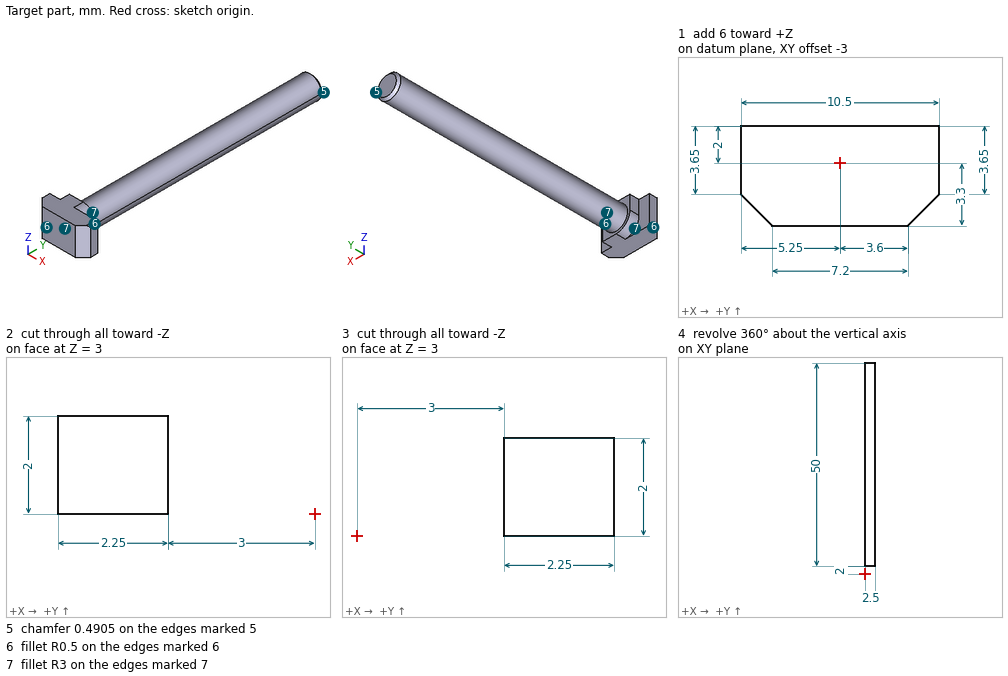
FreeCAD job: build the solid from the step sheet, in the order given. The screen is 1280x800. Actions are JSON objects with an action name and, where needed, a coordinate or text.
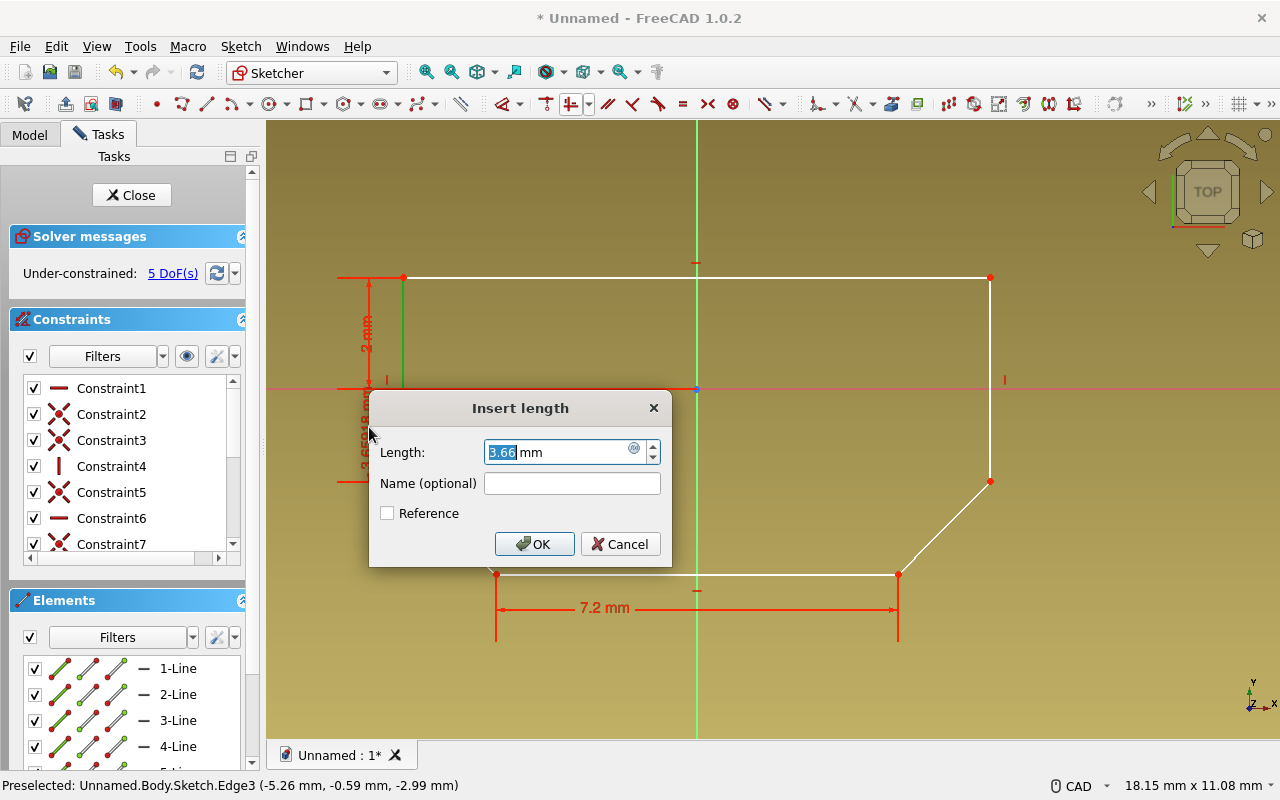
{"action": "type", "text": "3.65"}
{"action": "key", "text": "Return"}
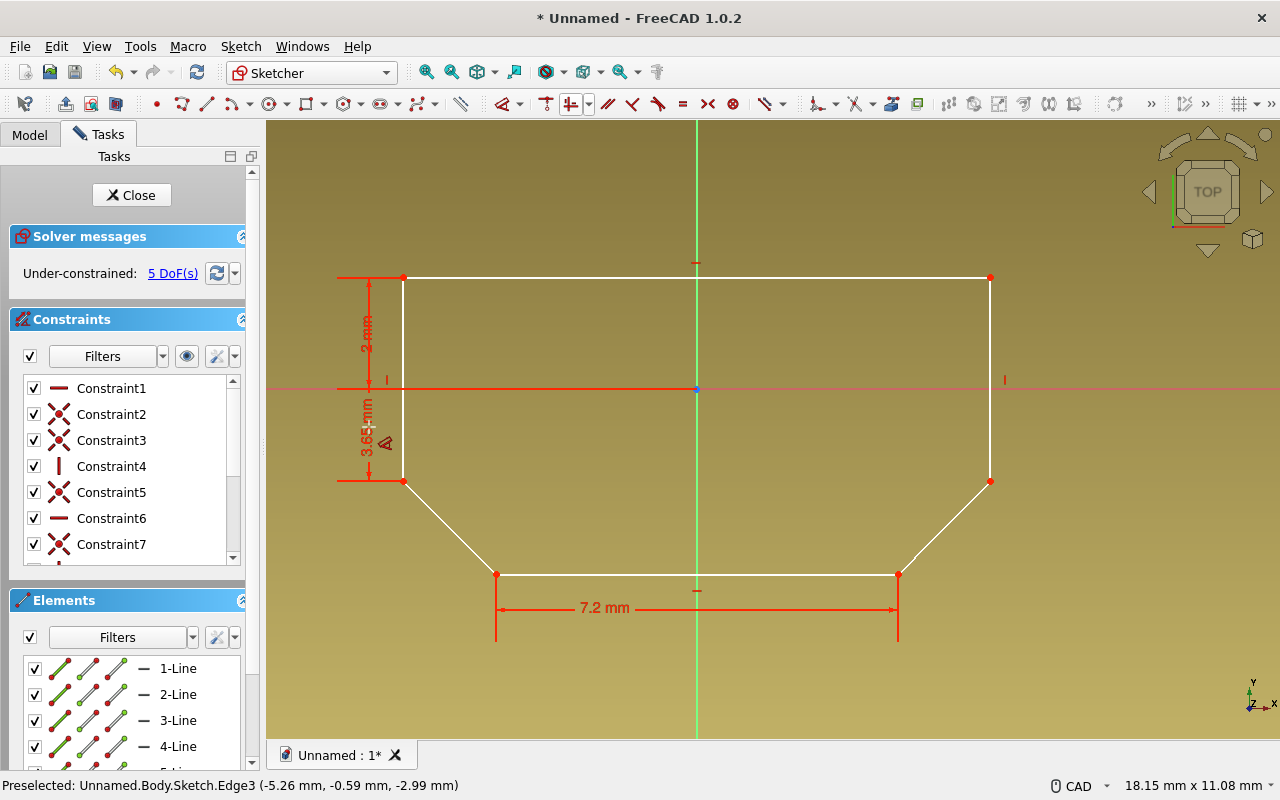
{"action": "left_click", "coordinate": [579, 278]}
{"action": "left_click", "coordinate": [561, 244]}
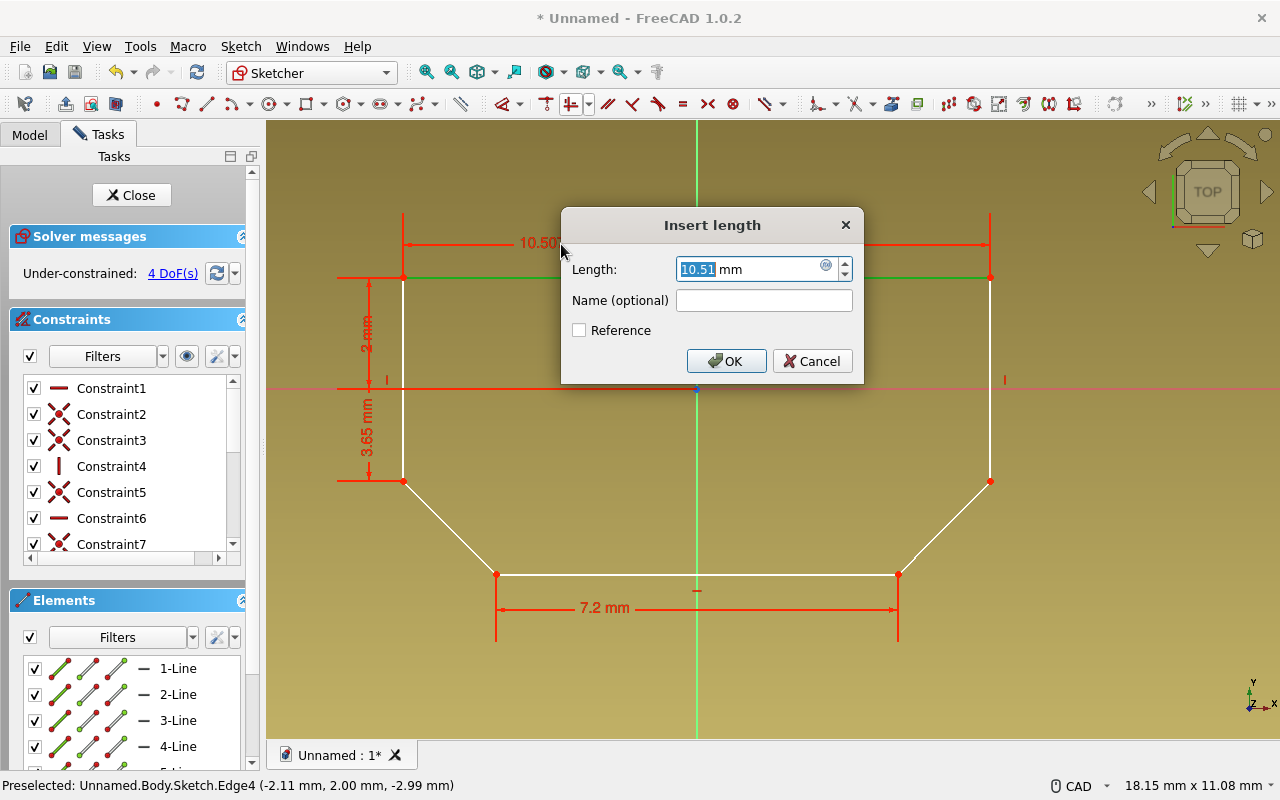
{"action": "type", "text": "10.5"}
{"action": "key", "text": "Return"}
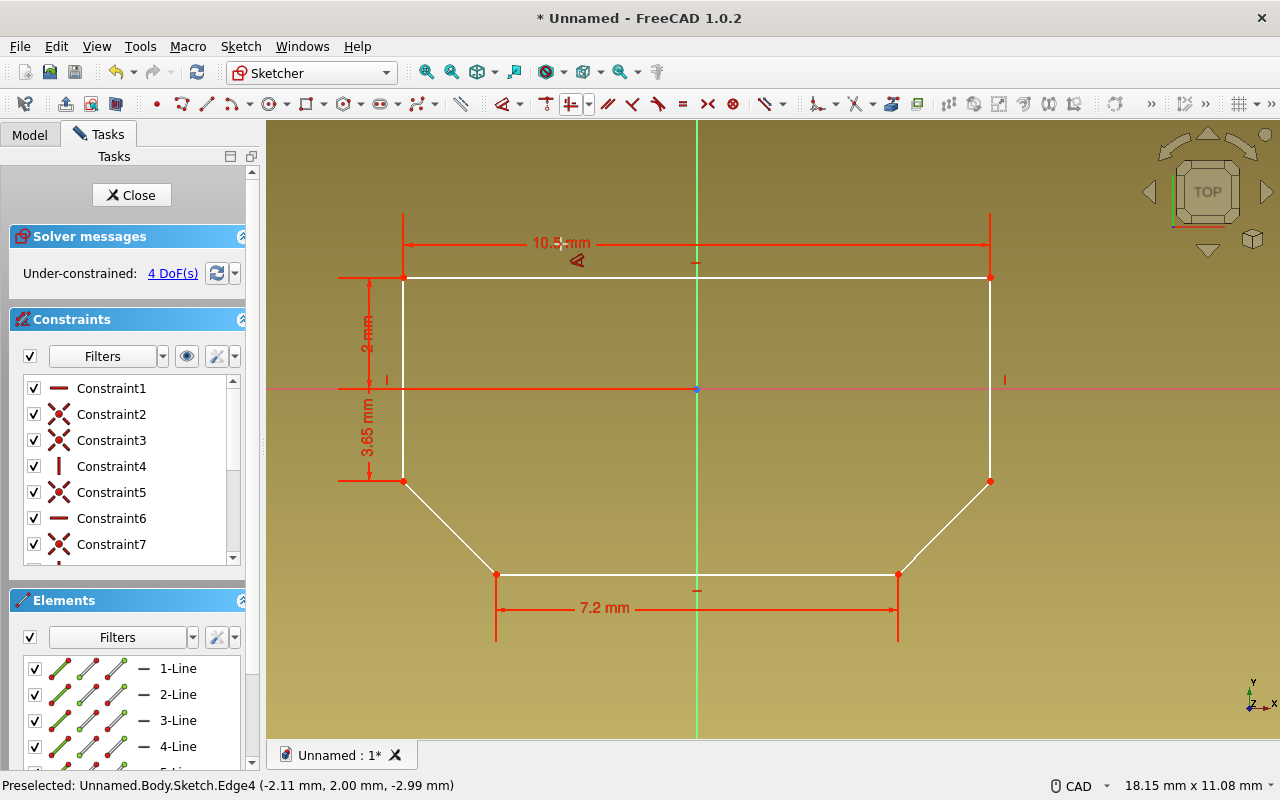
{"action": "left_click", "coordinate": [990, 339]}
{"action": "left_click", "coordinate": [1024, 333]}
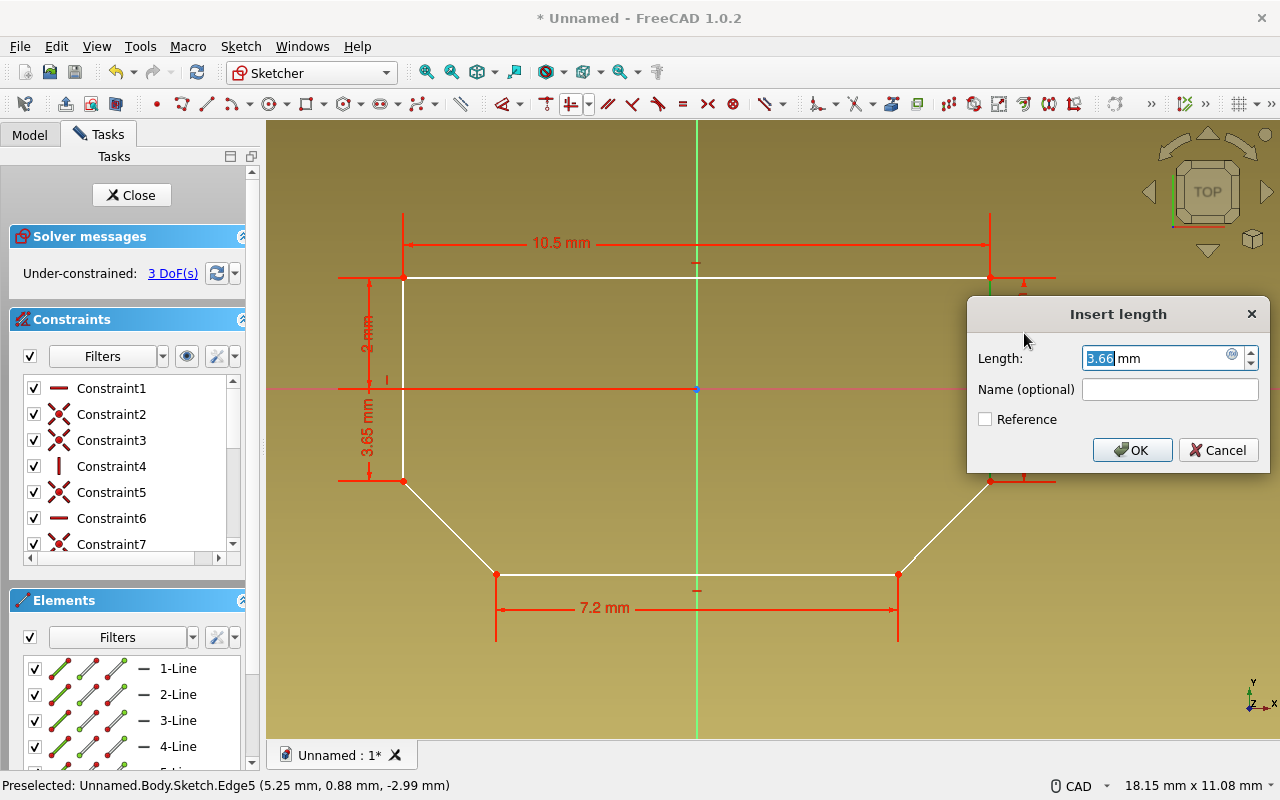
{"action": "type", "text": "3.65"}
{"action": "key", "text": "Return"}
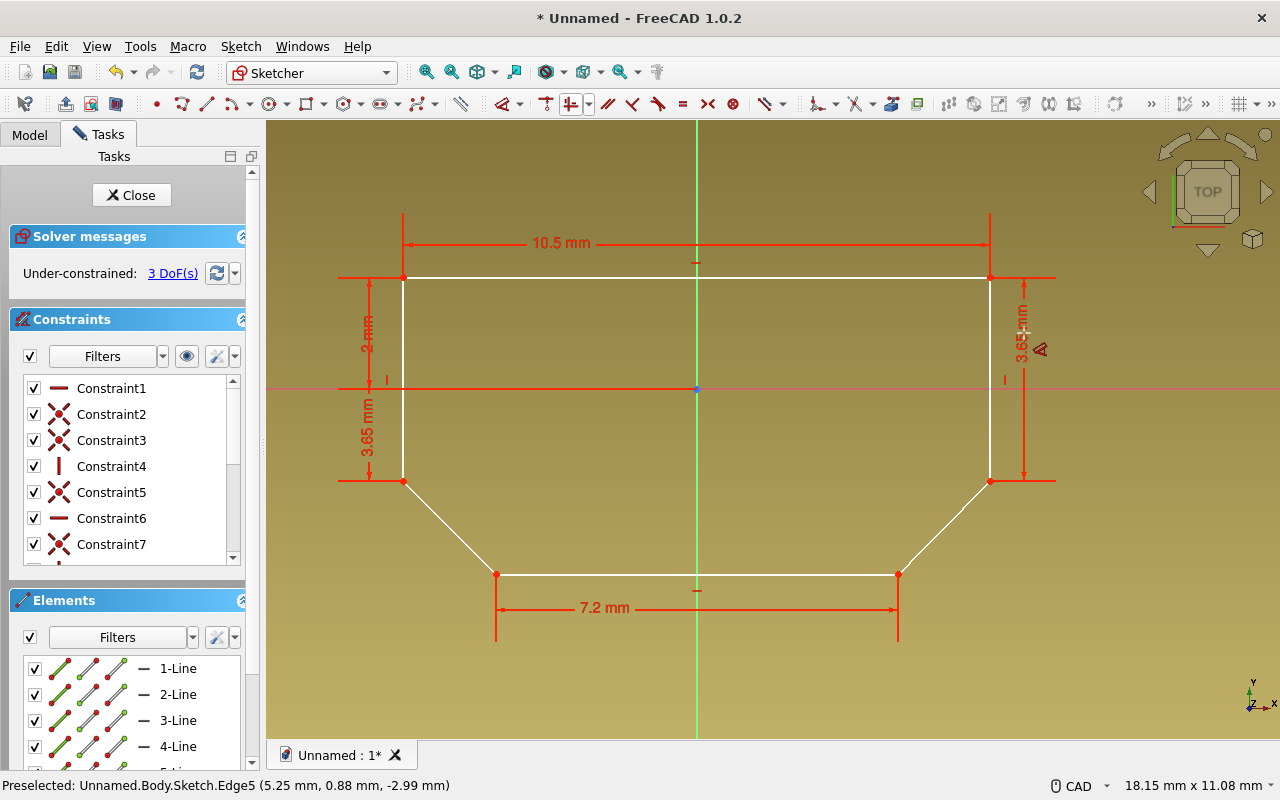
{"action": "left_click", "coordinate": [898, 575]}
{"action": "left_click", "coordinate": [797, 609]}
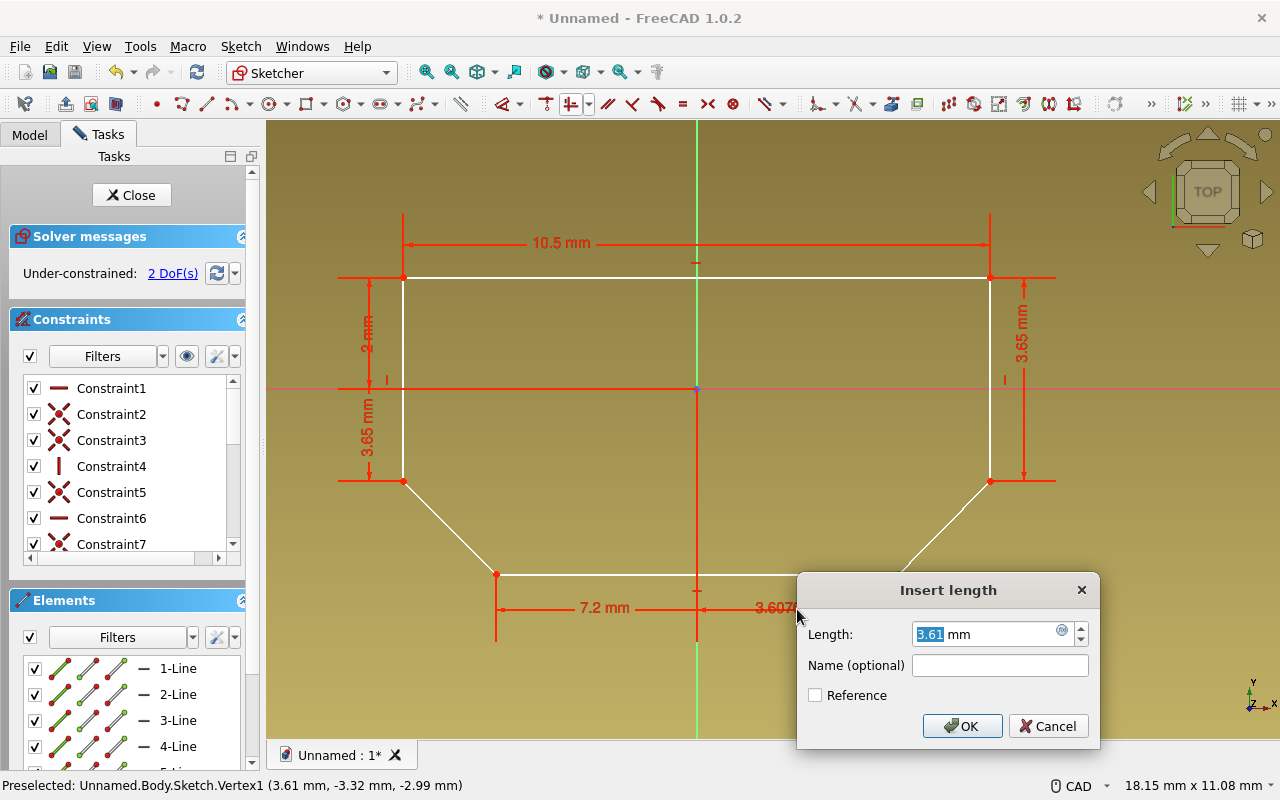
{"action": "type", "text": "3.6"}
{"action": "key", "text": "Return"}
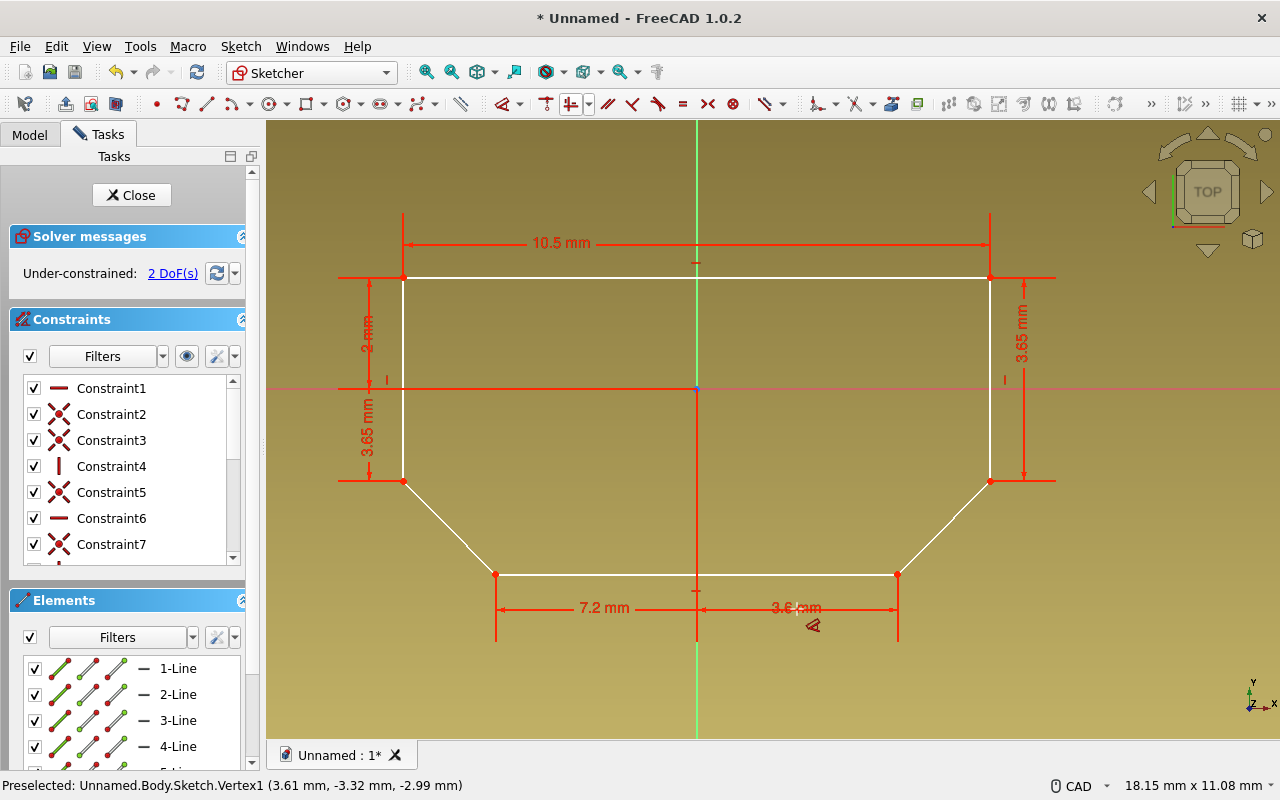
{"action": "left_click", "coordinate": [898, 575]}
{"action": "left_click", "coordinate": [932, 482]}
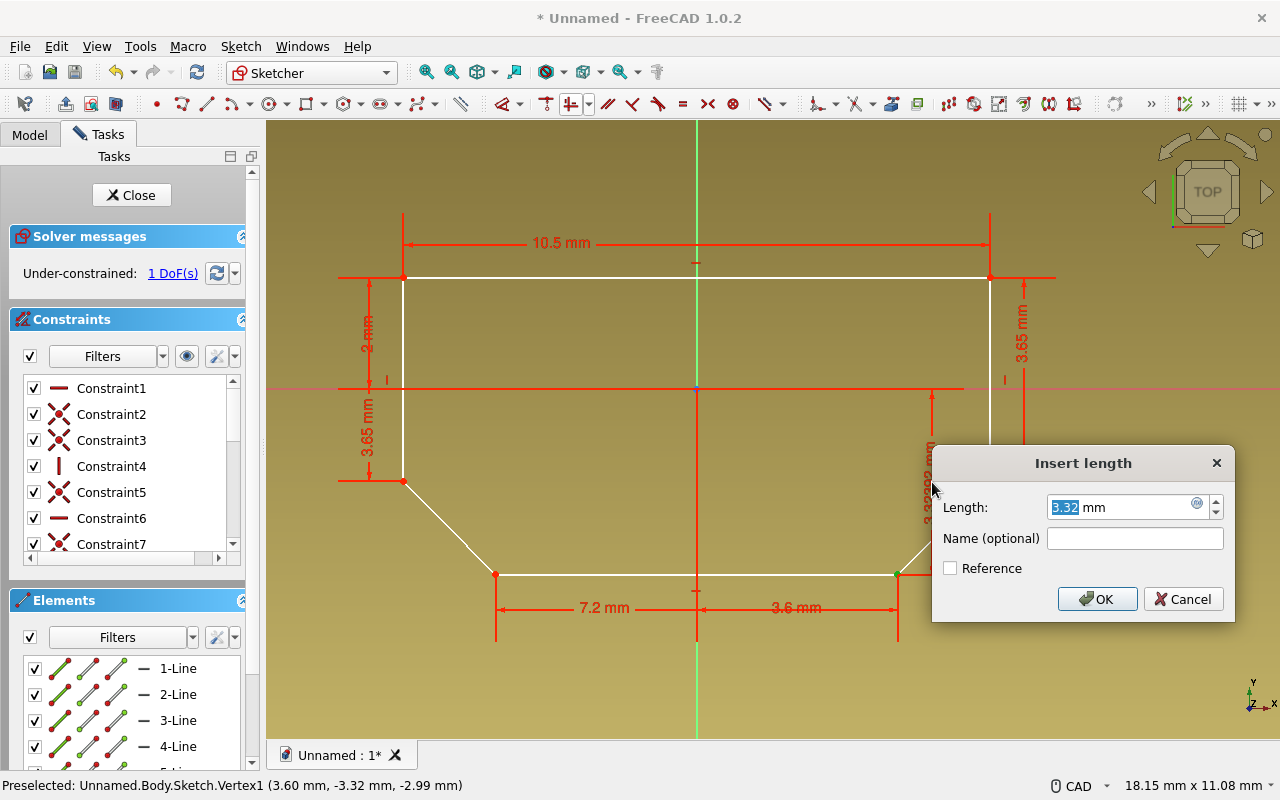
{"action": "type", "text": "3.3"}
{"action": "key", "text": "Return"}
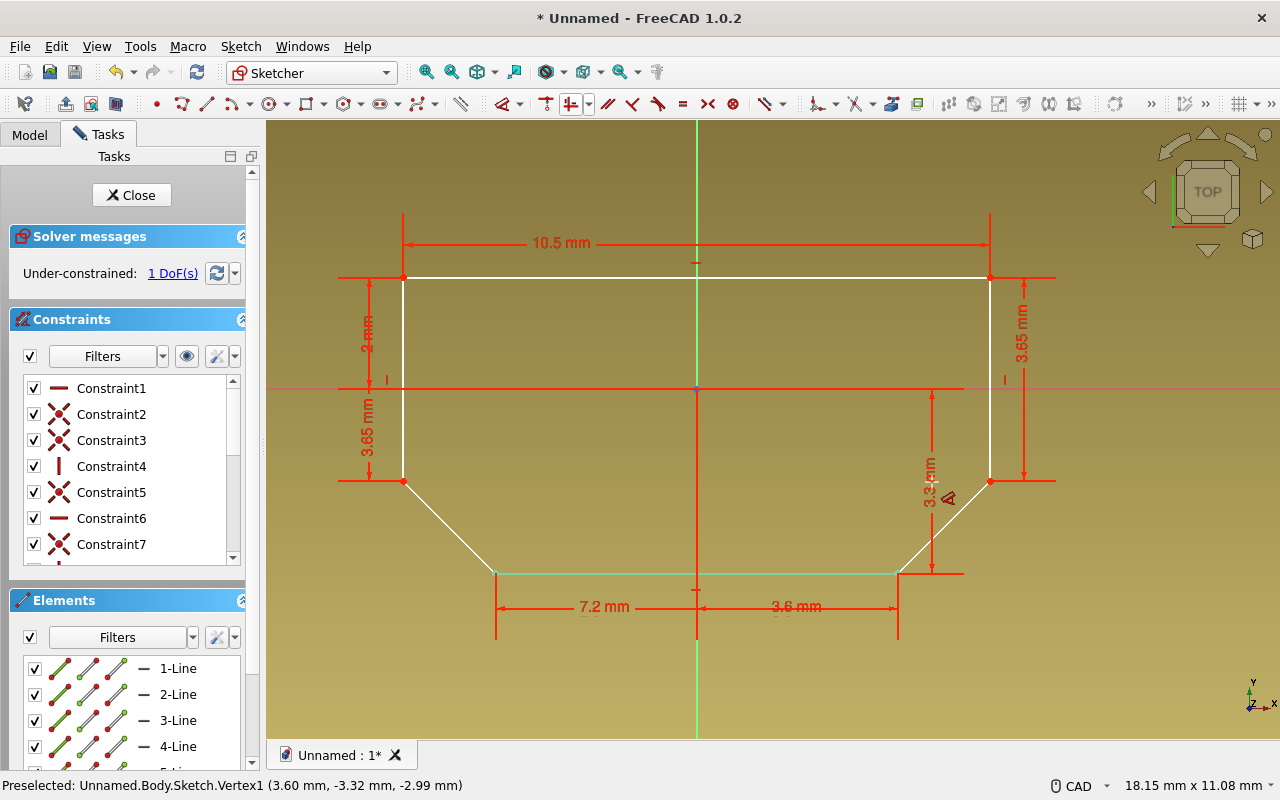
{"action": "left_click", "coordinate": [403, 481]}
{"action": "left_click", "coordinate": [550, 515]}